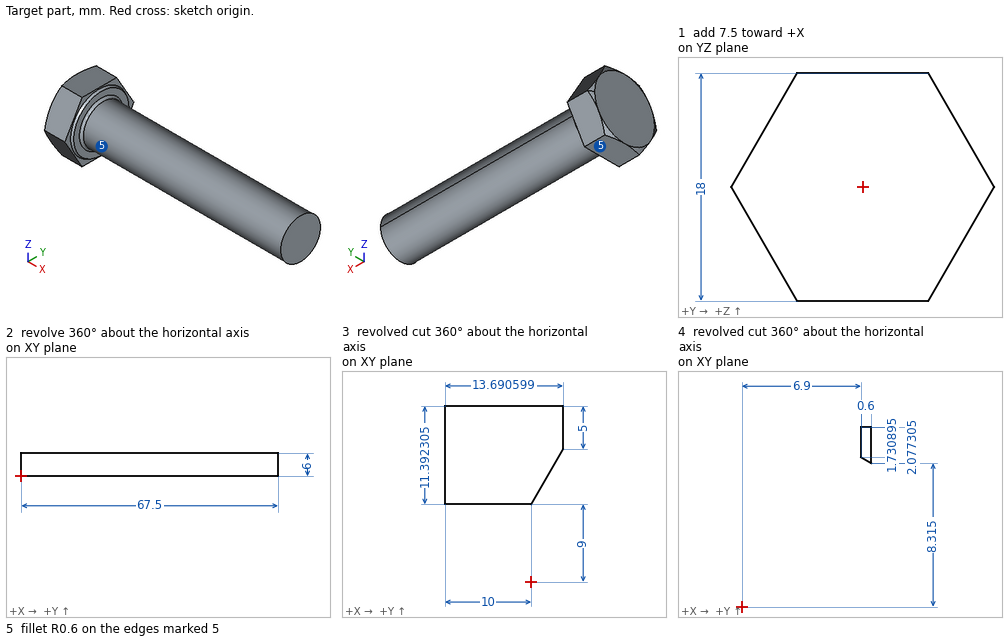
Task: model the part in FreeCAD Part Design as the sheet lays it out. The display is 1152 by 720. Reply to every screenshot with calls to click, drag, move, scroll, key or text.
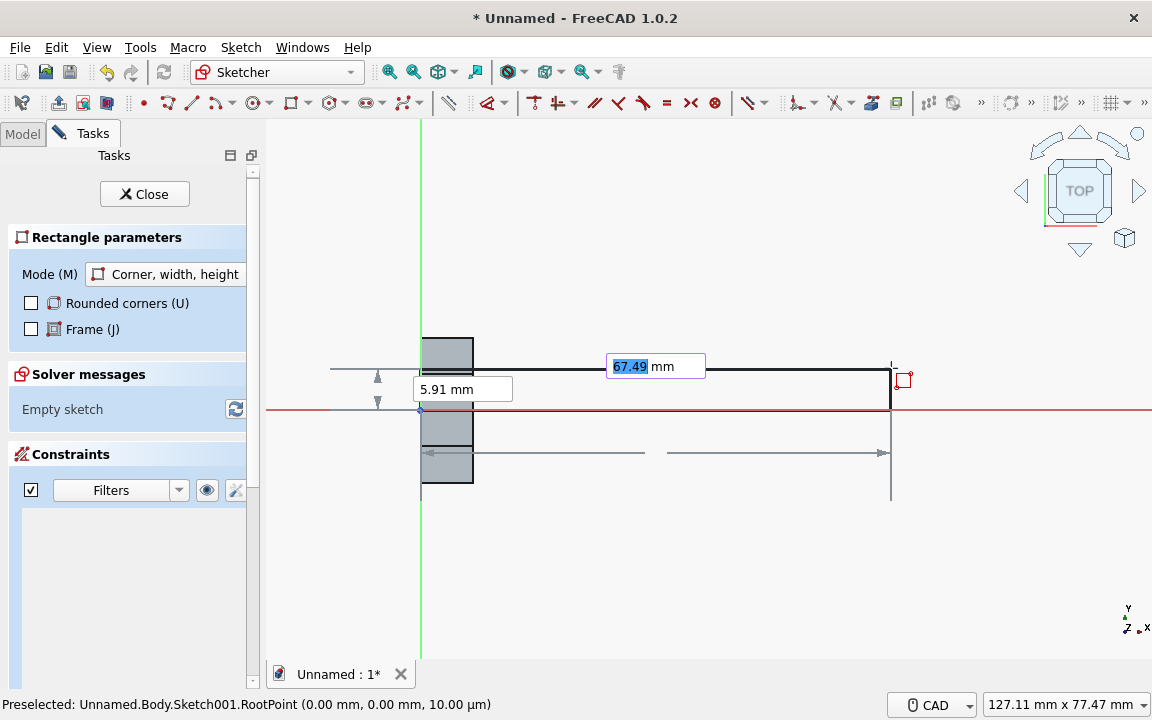
text(67.5)
key(Tab)
text(6)
key(Return)
key(Escape)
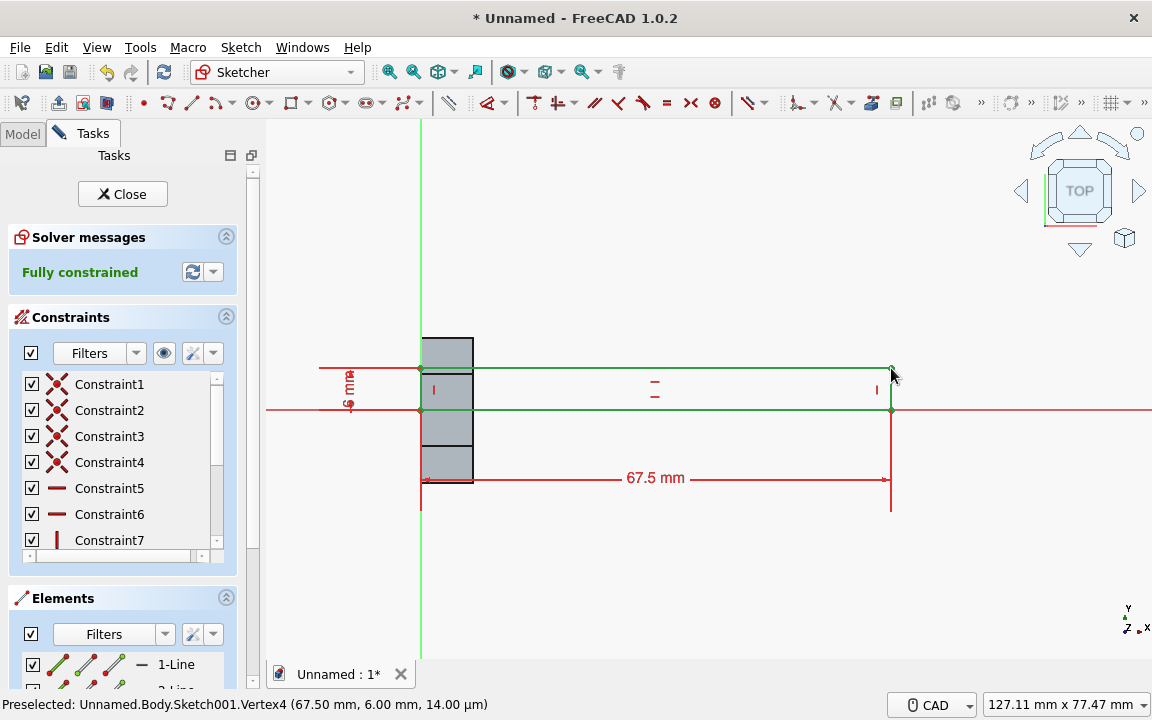
click(123, 194)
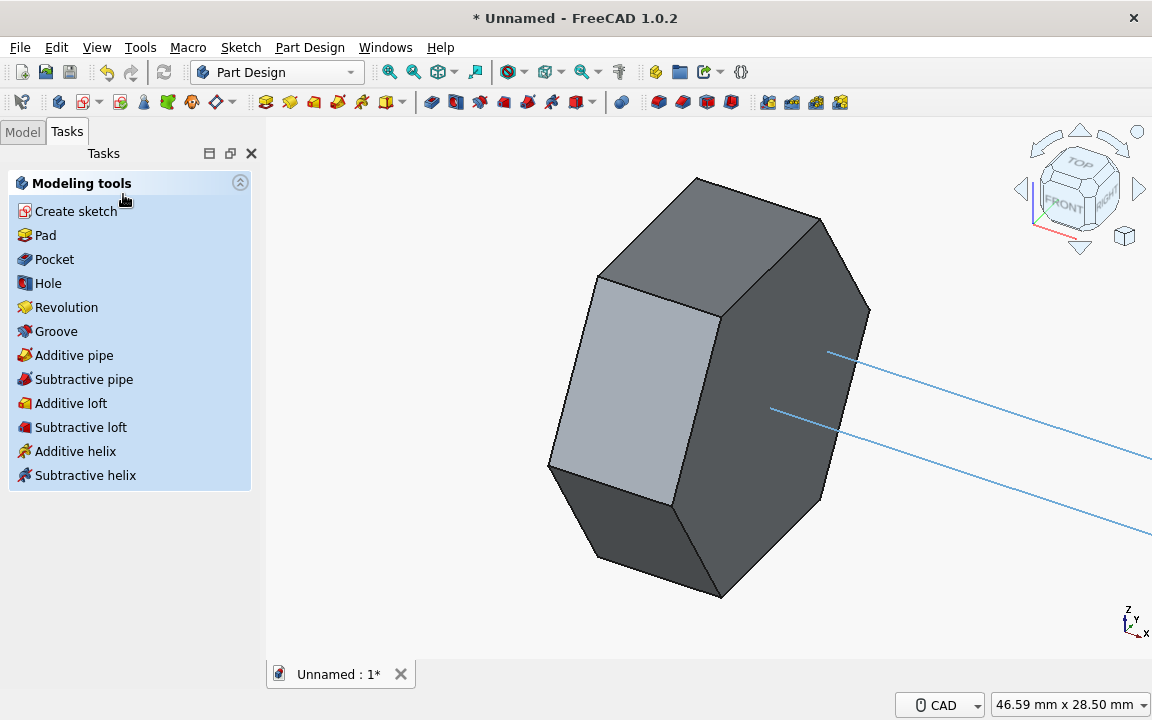
click(290, 102)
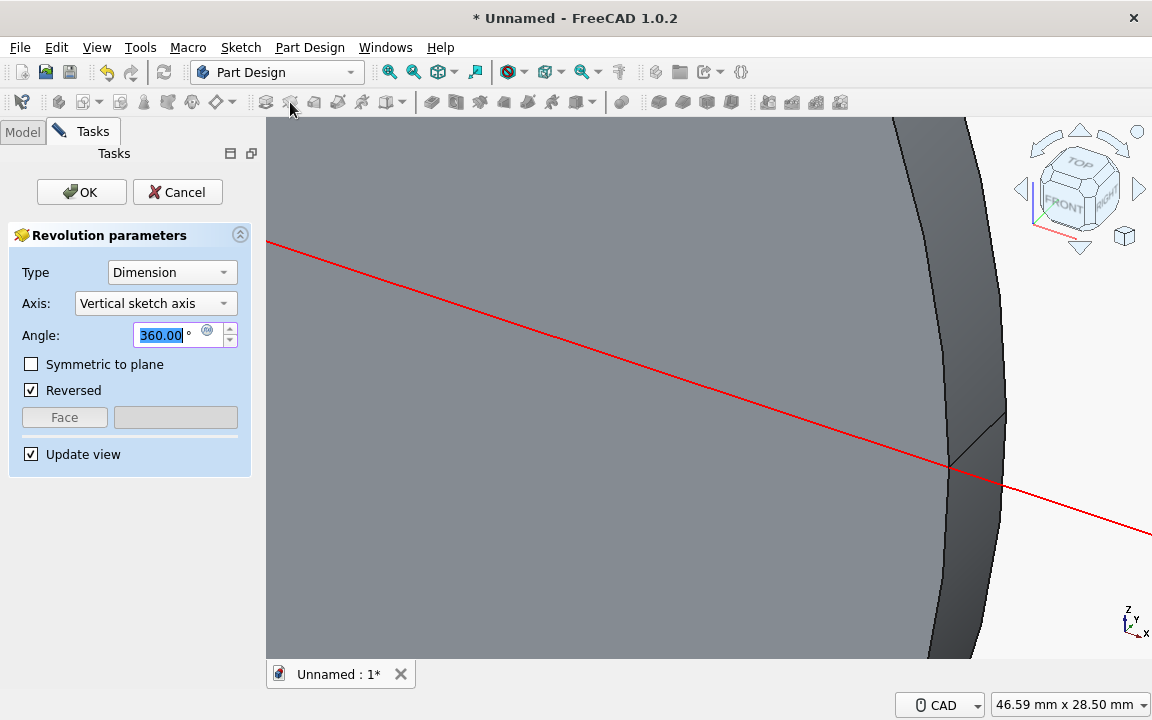
click(156, 304)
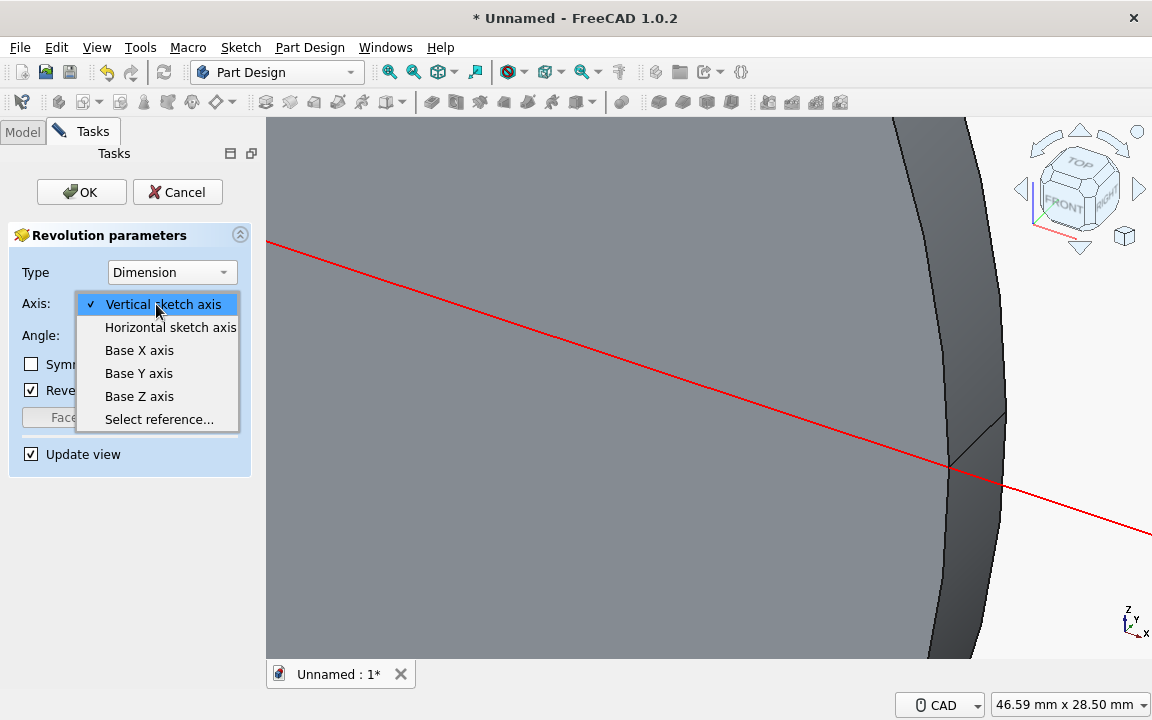
click(156, 328)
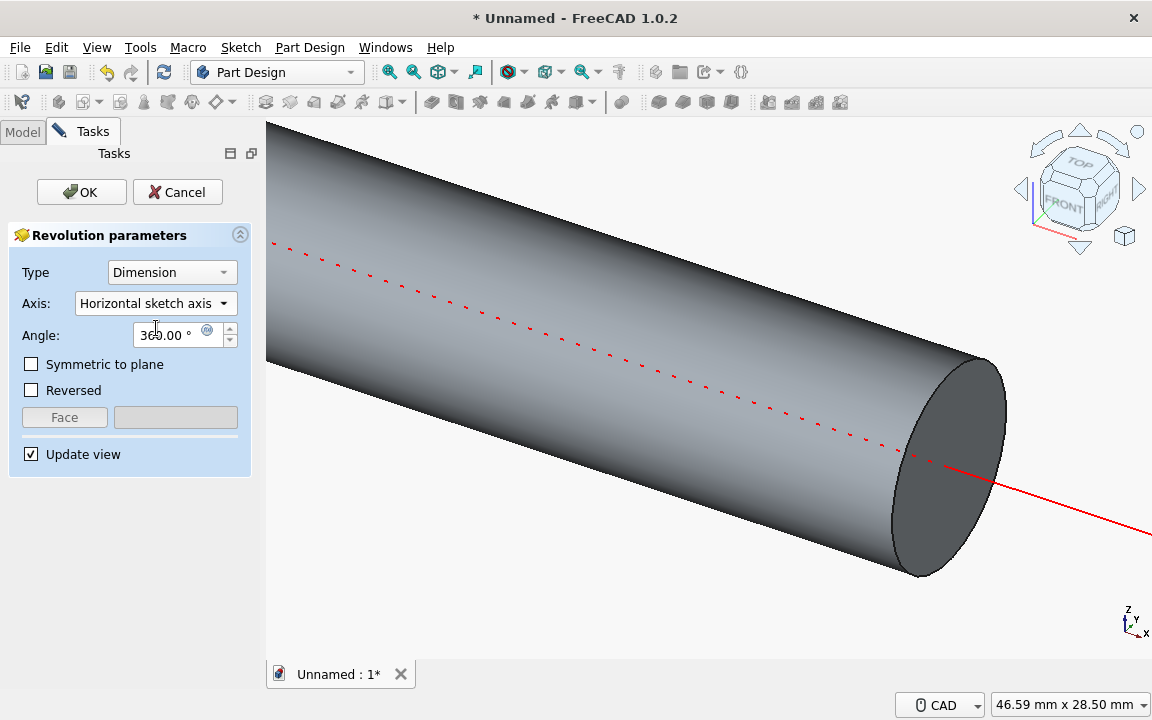
click(82, 192)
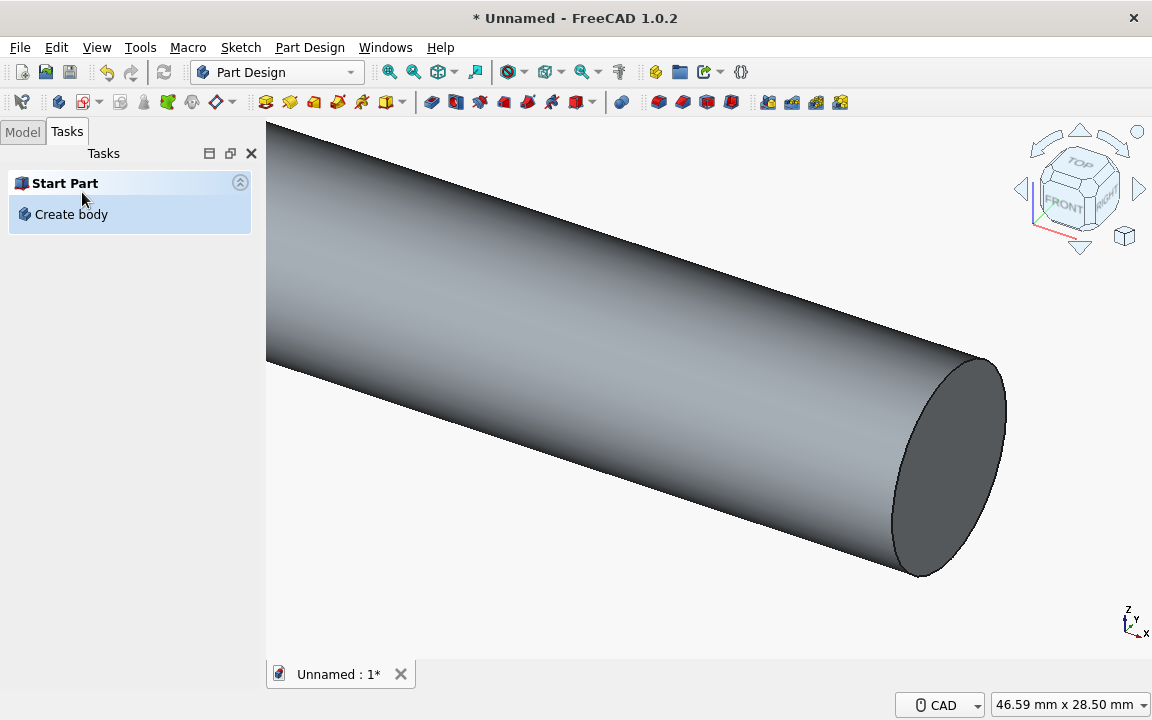
key(v)
key(f)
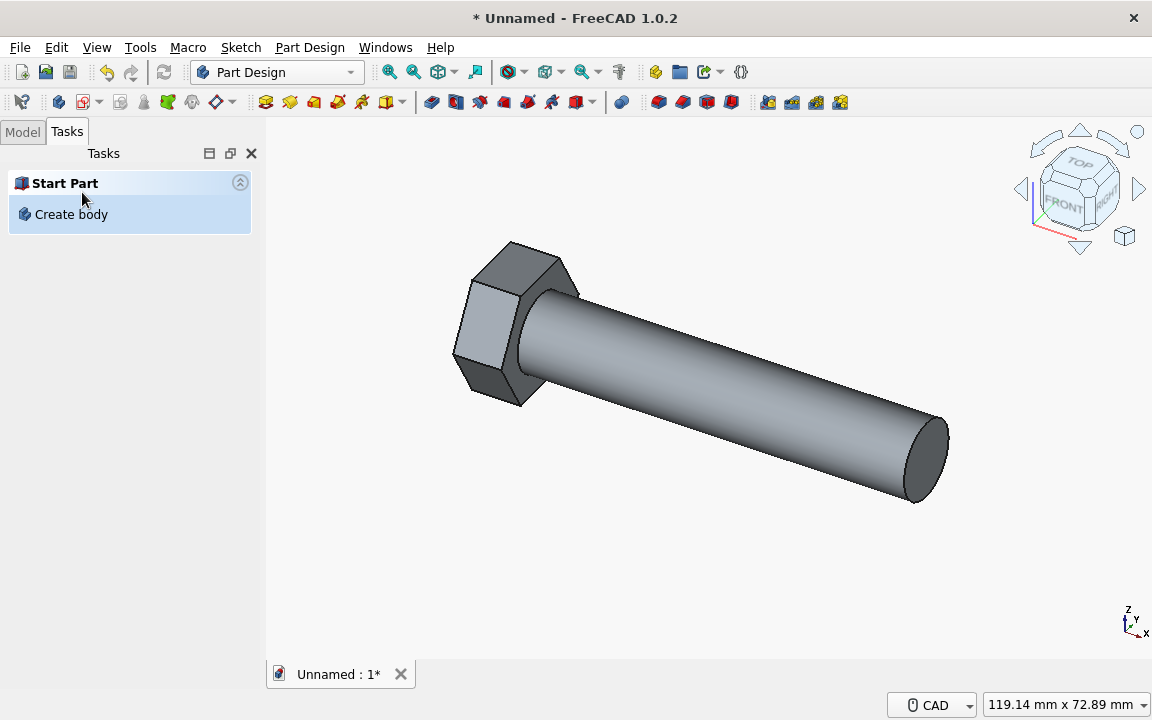
click(84, 102)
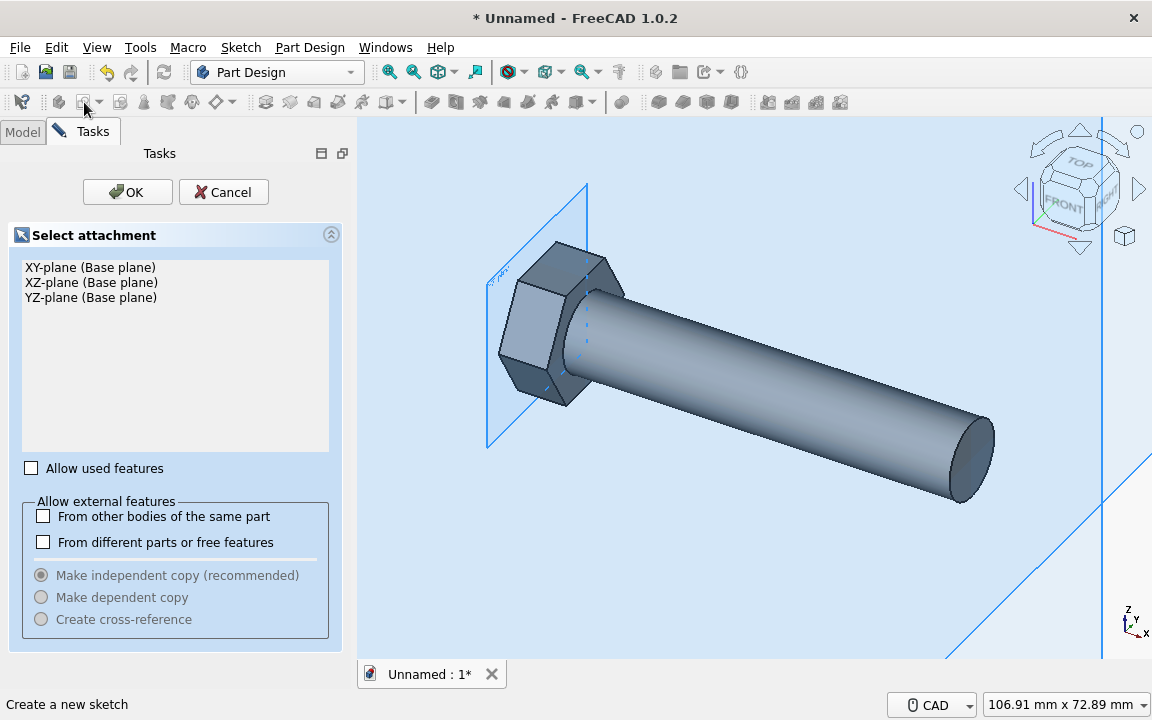
click(82, 268)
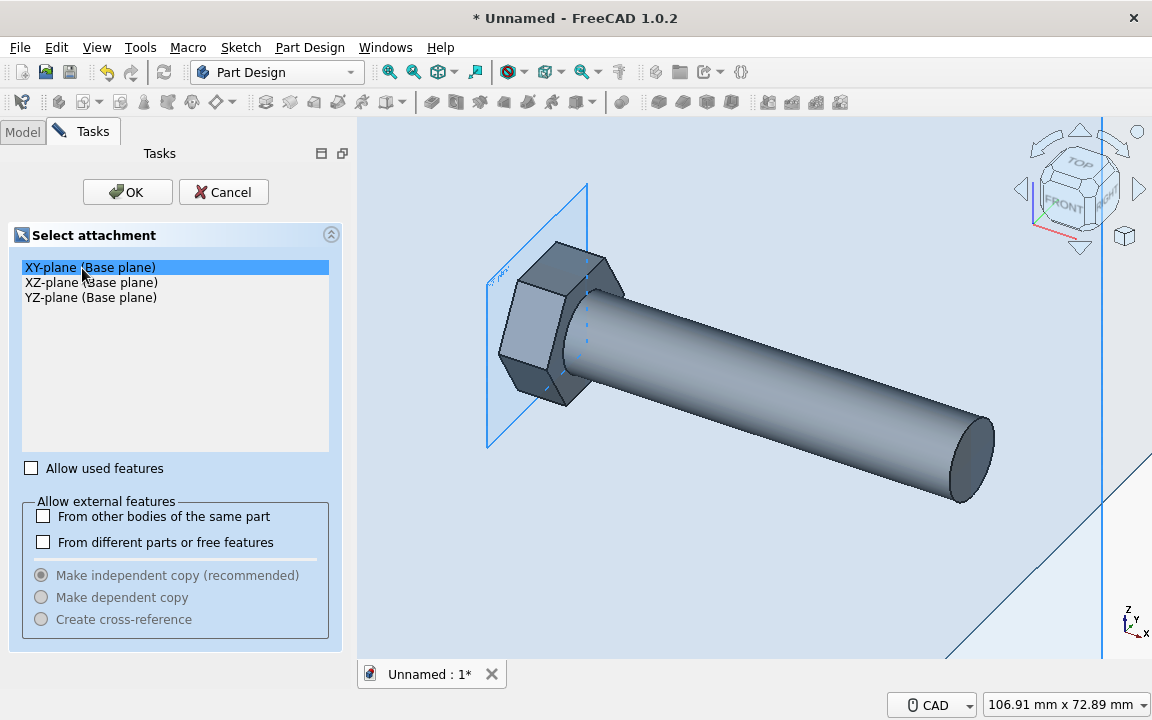
click(128, 192)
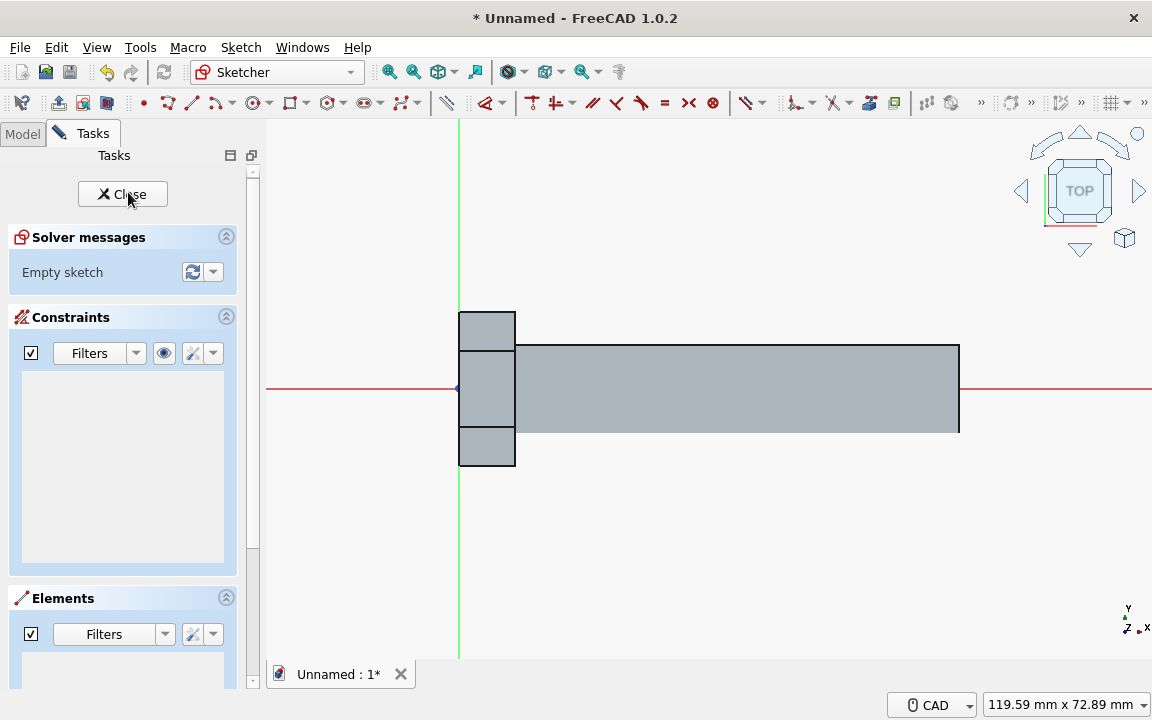
key(q)
key(s)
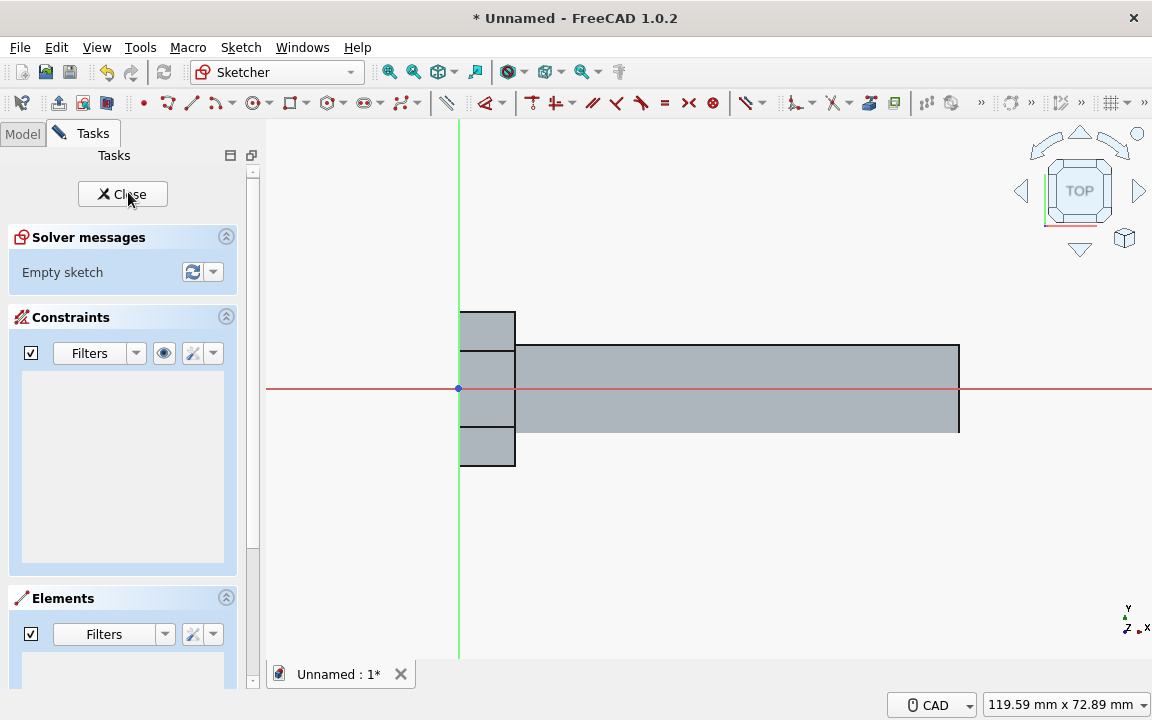
scroll(294, 252, up, 4)